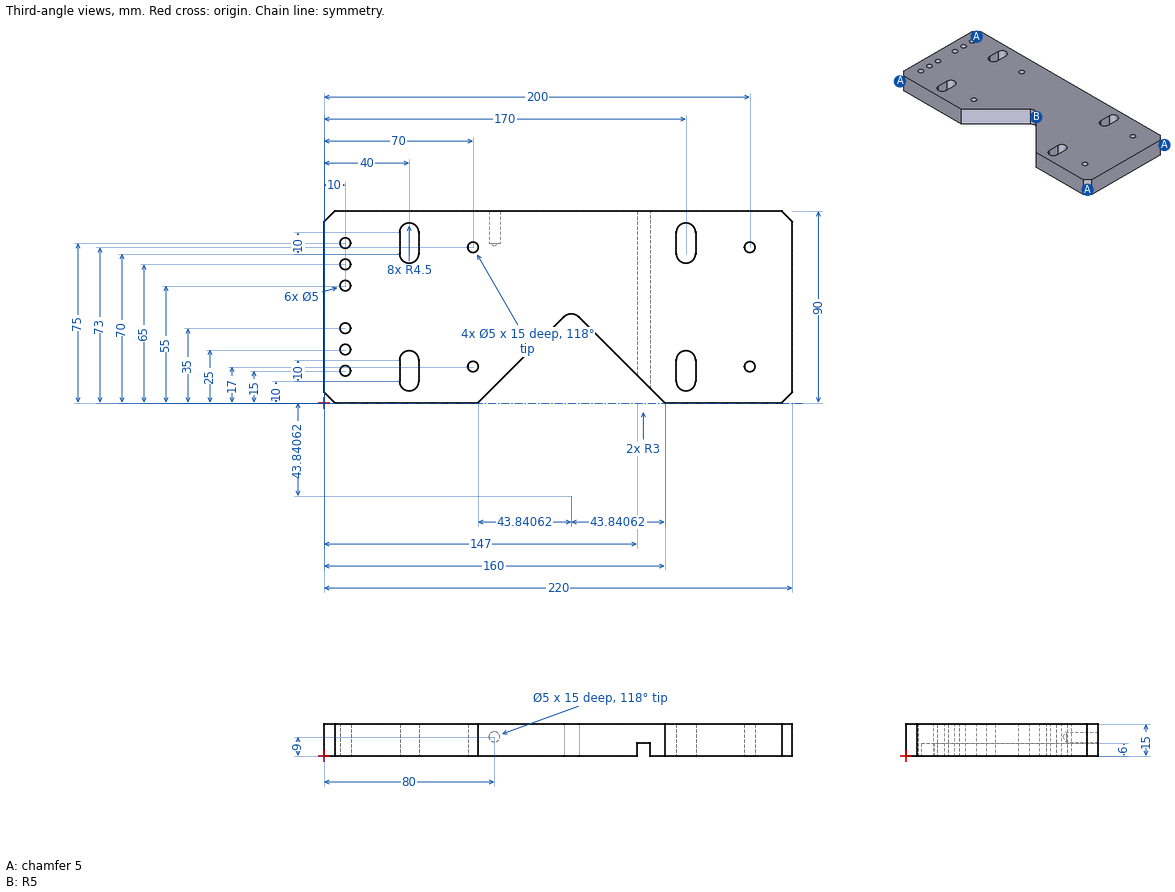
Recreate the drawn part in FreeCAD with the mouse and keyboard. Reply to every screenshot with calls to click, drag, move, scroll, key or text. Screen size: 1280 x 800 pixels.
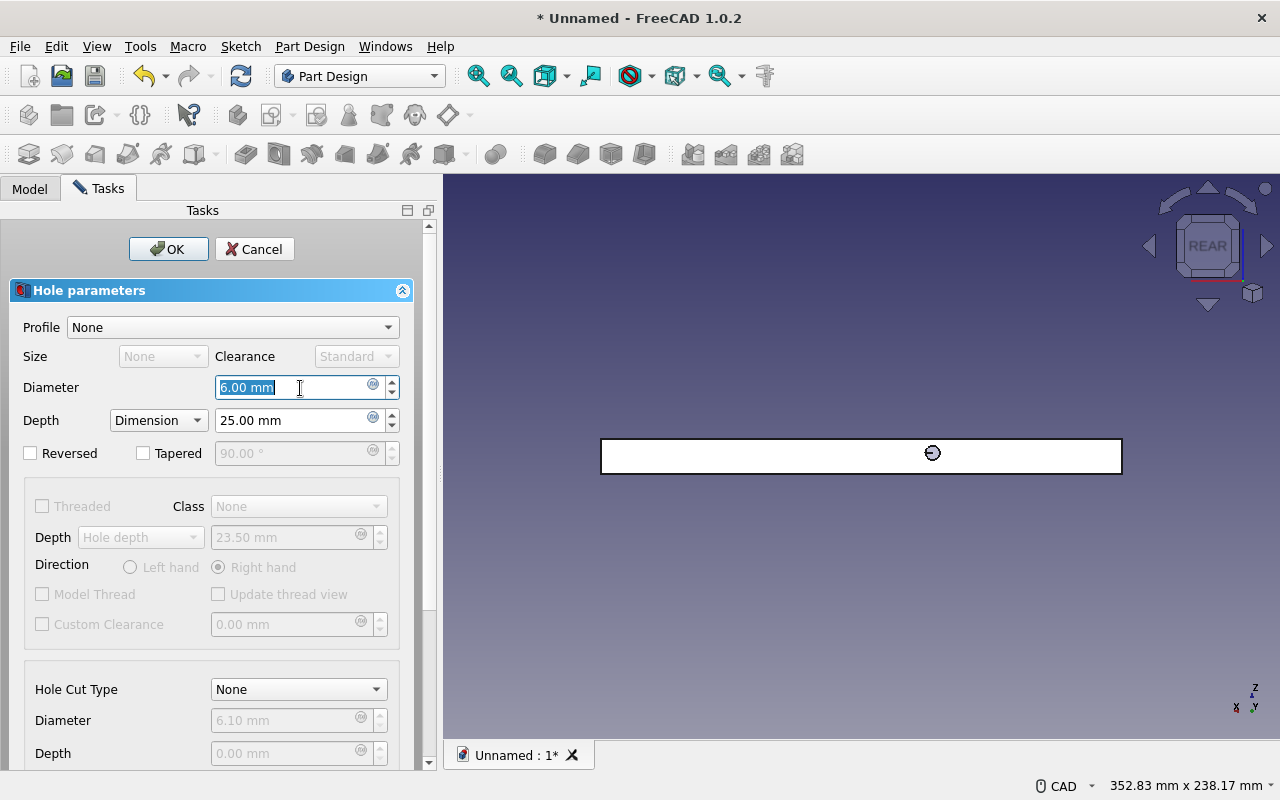
text(5)
key(Tab)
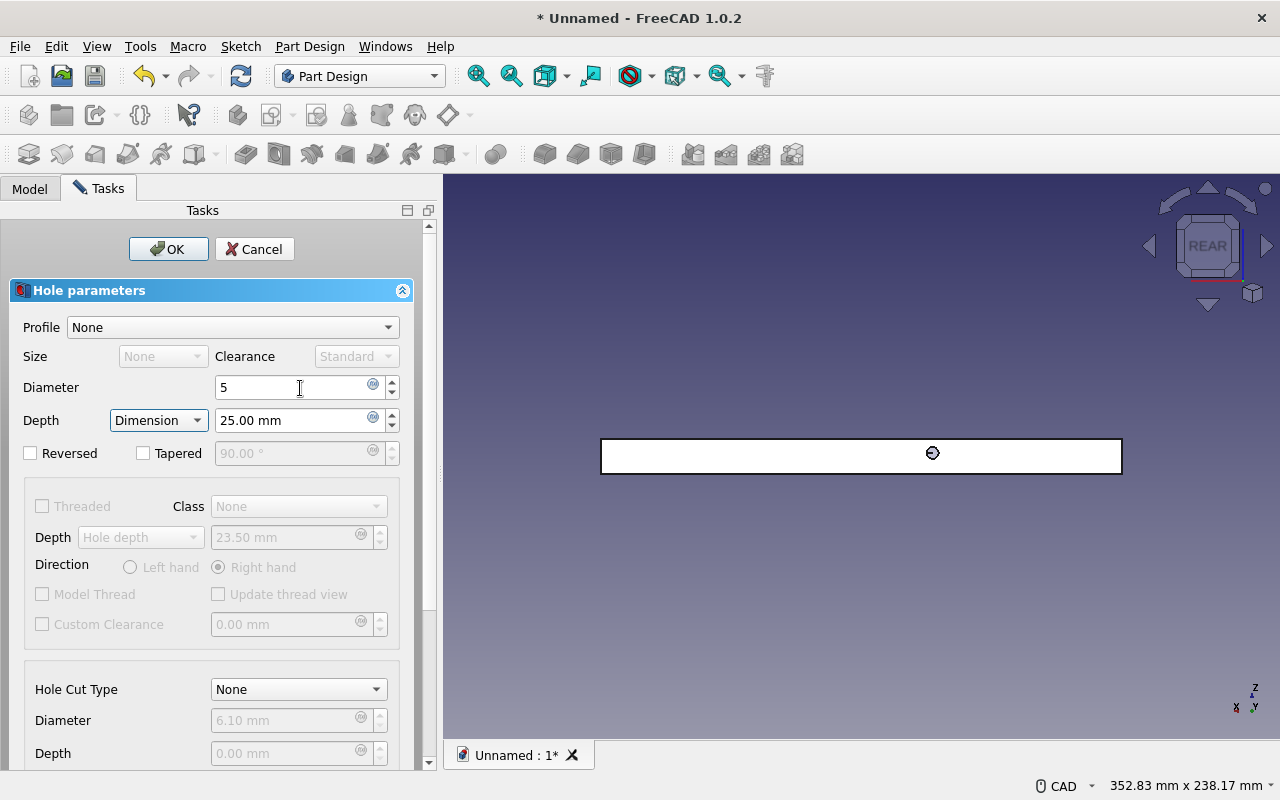
triple_click(300, 420)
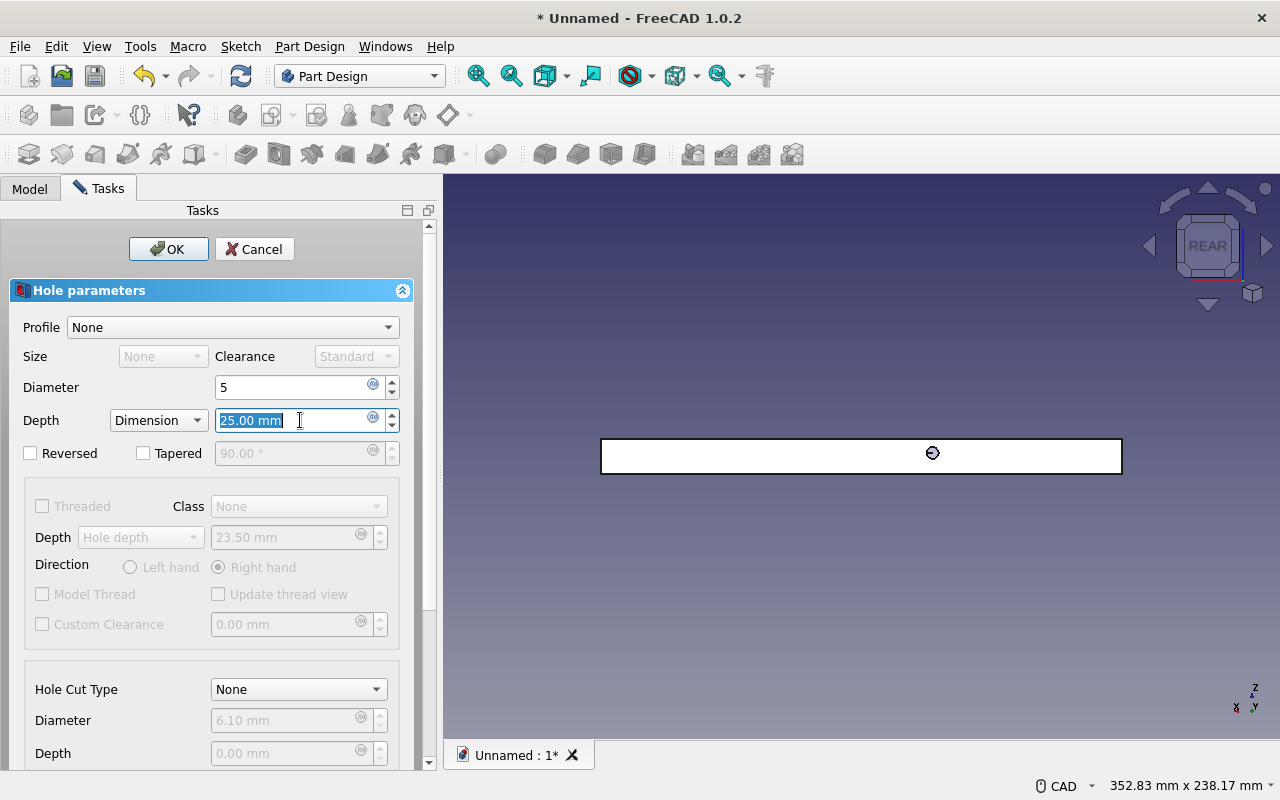
text(15)
key(Tab)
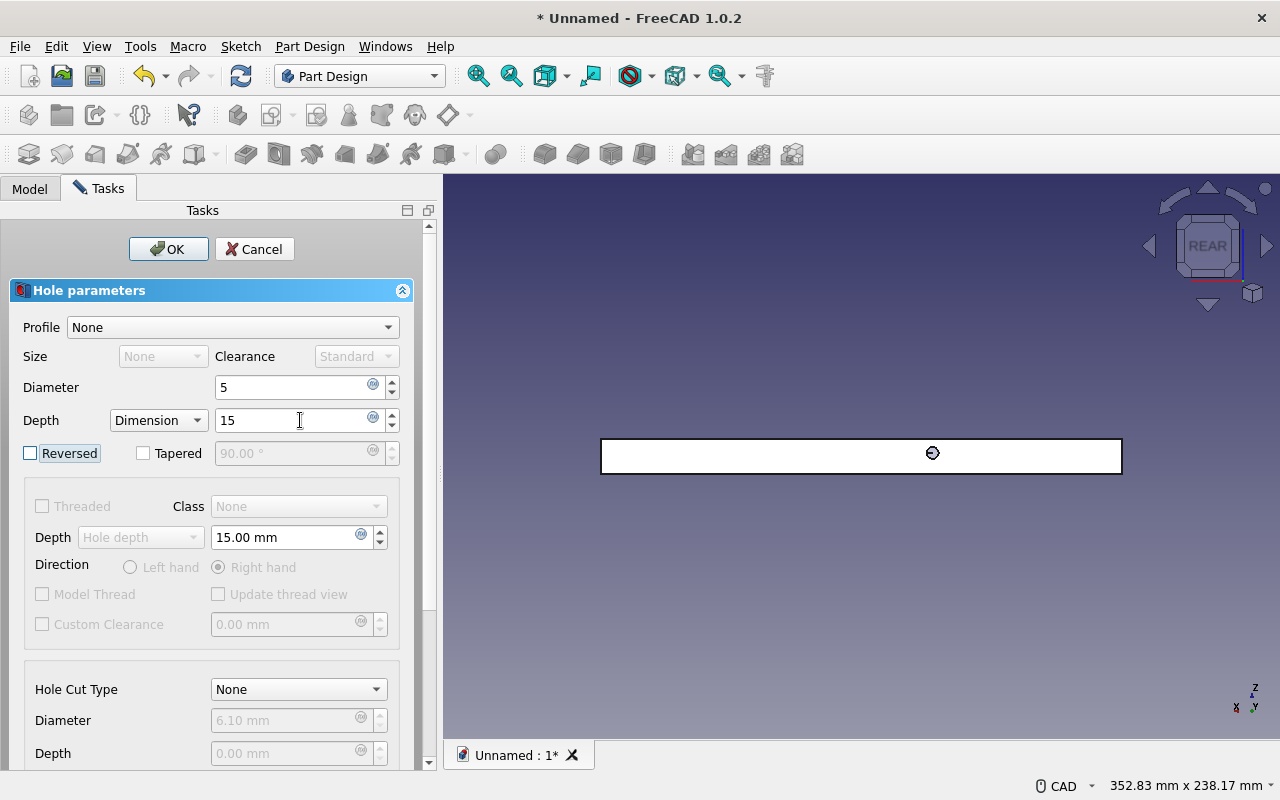
click(169, 249)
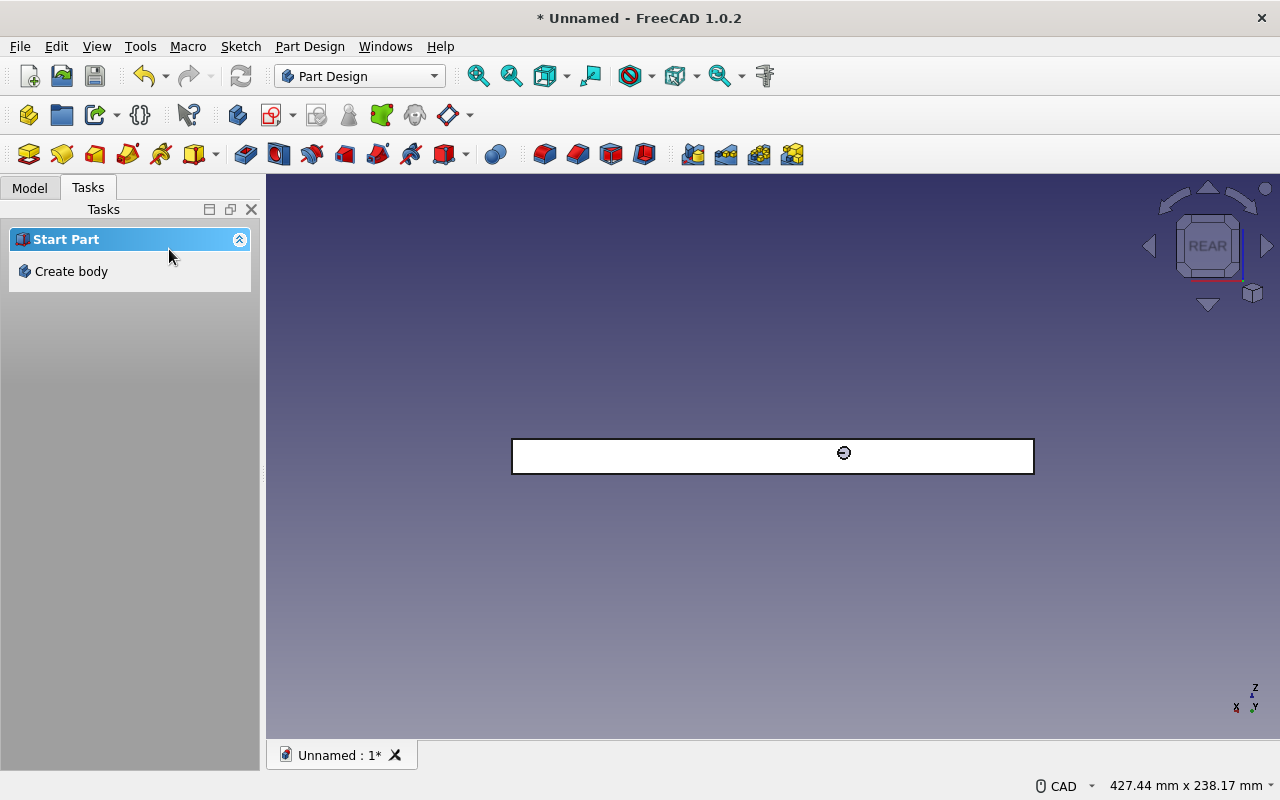
click(1034, 456)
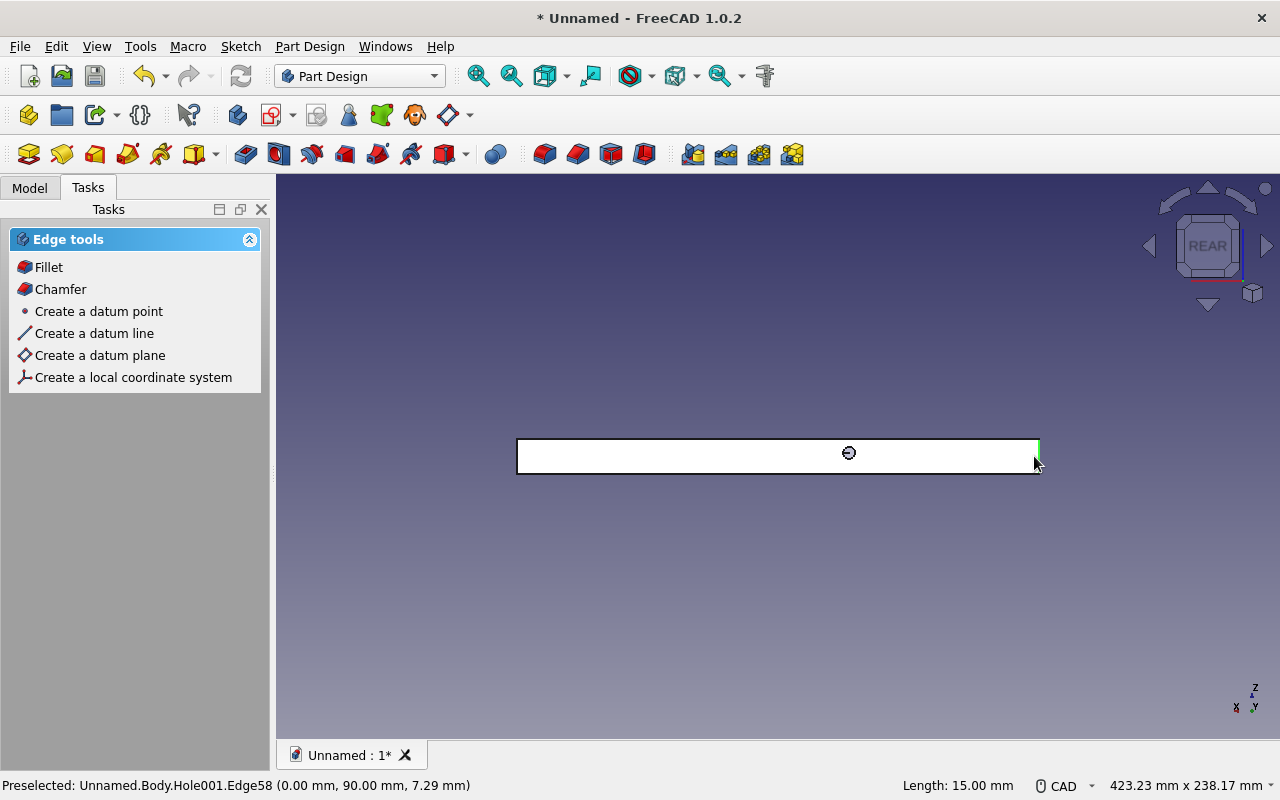
key(0)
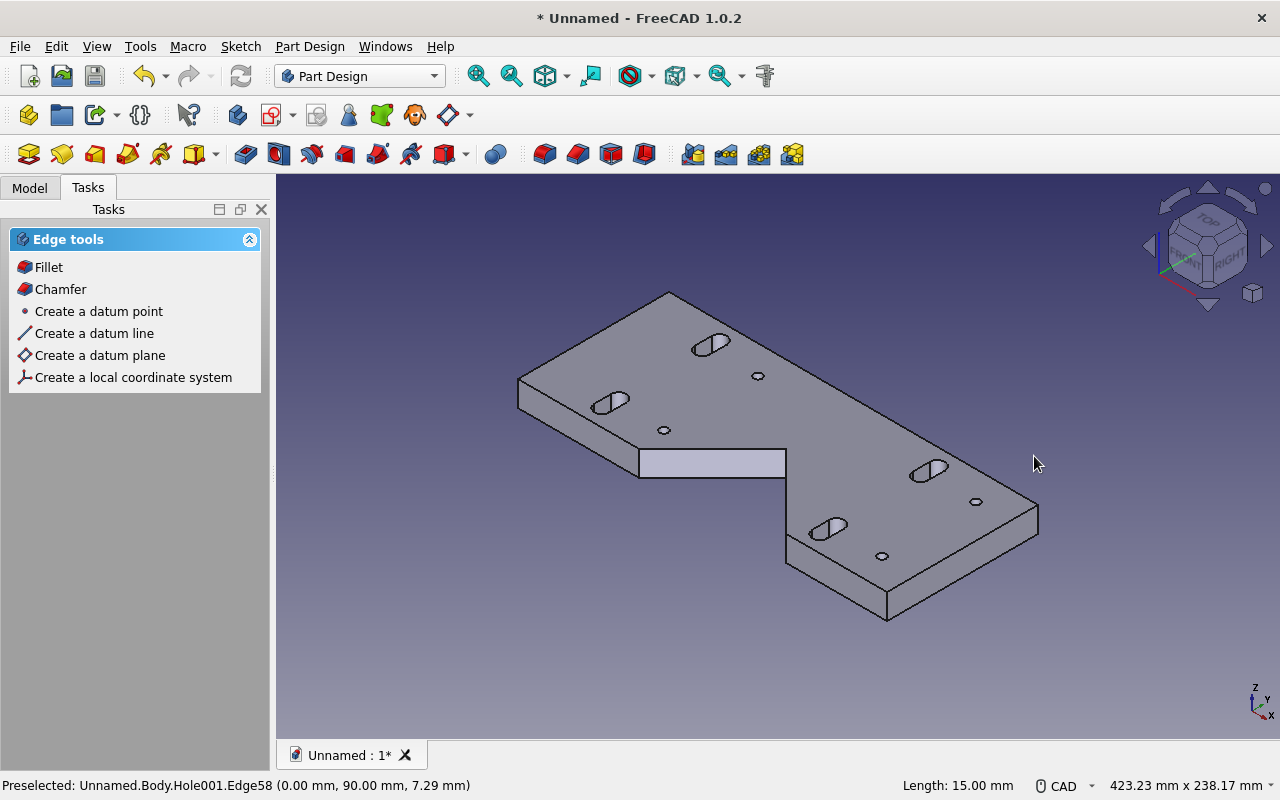
click(887, 606, ctrl)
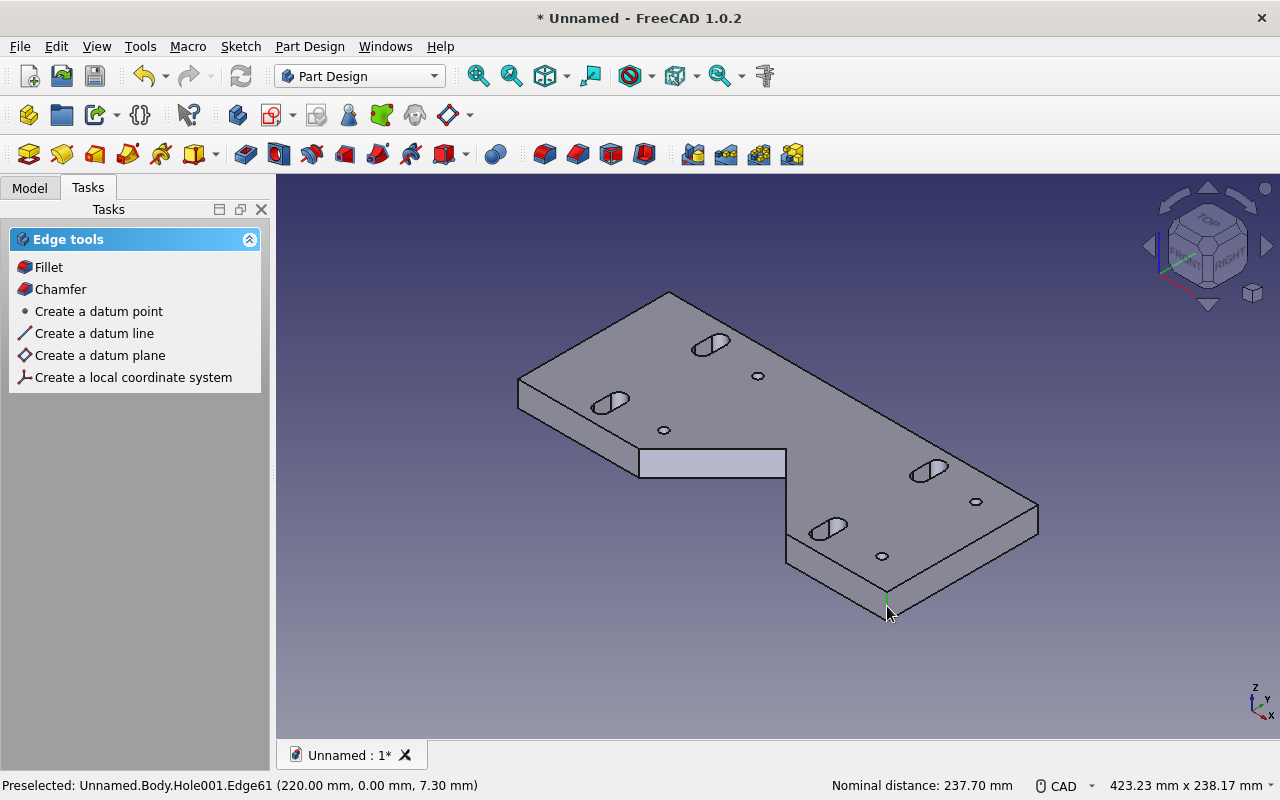
key(2)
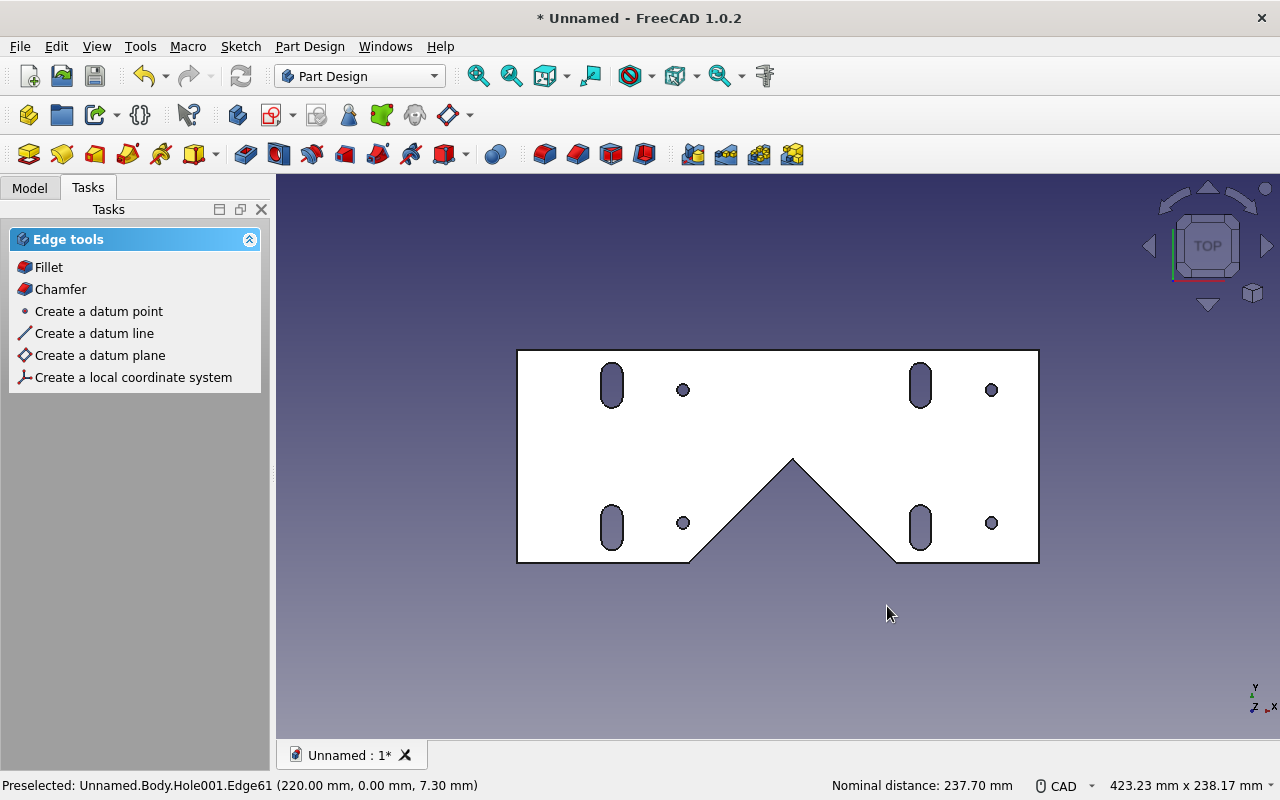
key(1)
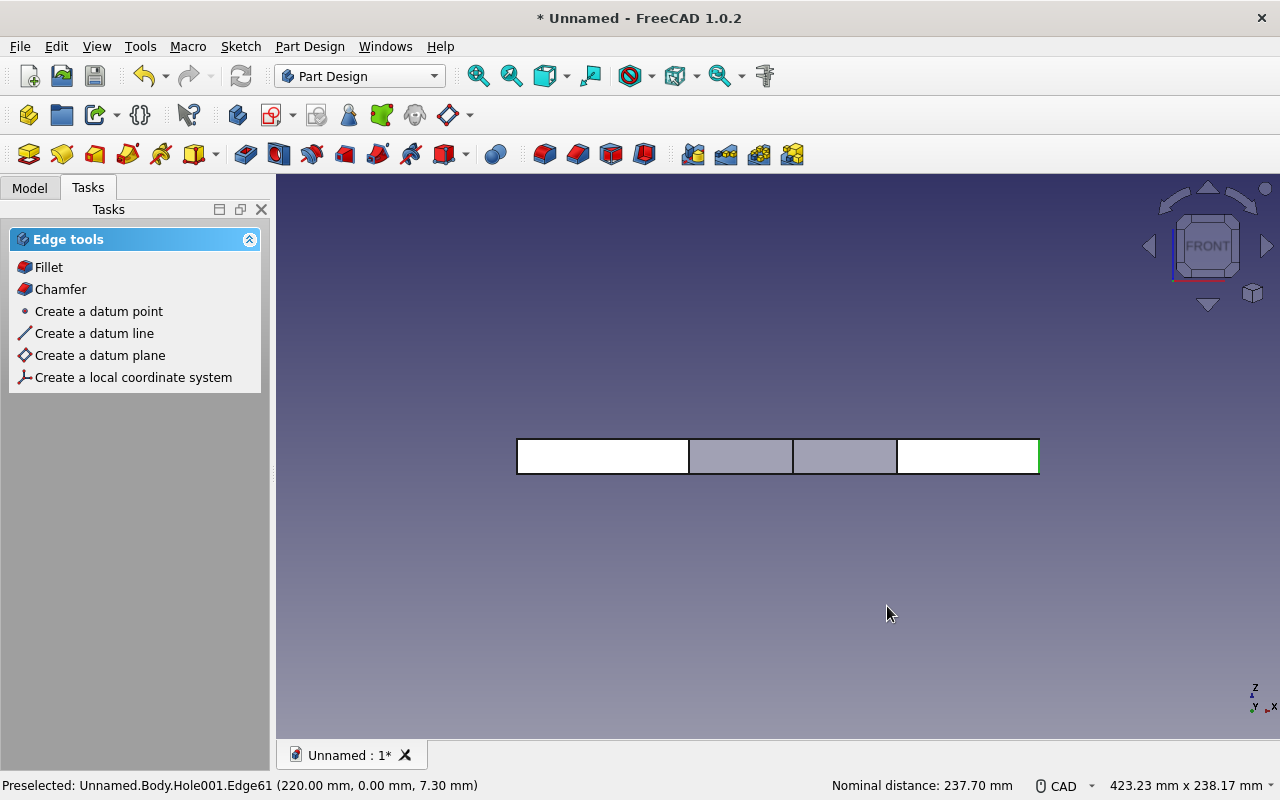
click(517, 456, ctrl)